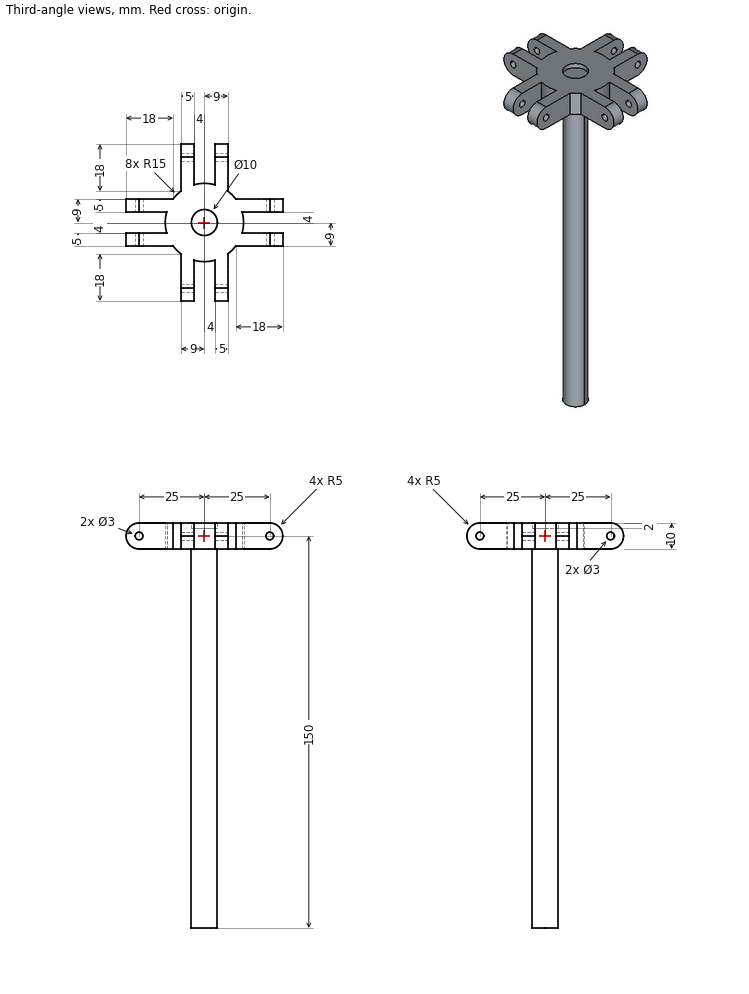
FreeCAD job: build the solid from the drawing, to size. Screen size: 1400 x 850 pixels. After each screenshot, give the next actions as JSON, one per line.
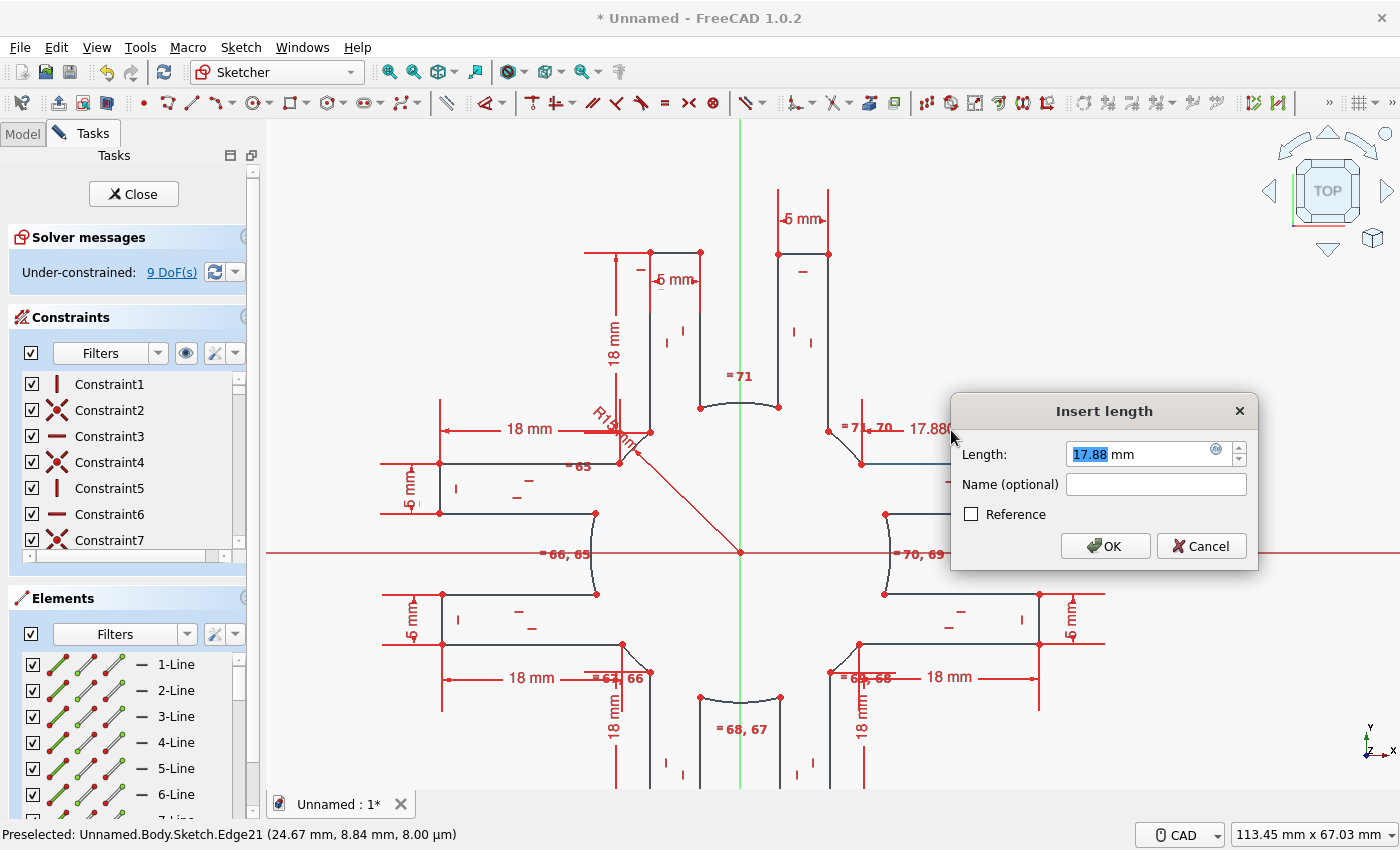
{"action": "type", "text": "18"}
{"action": "key", "text": "Return"}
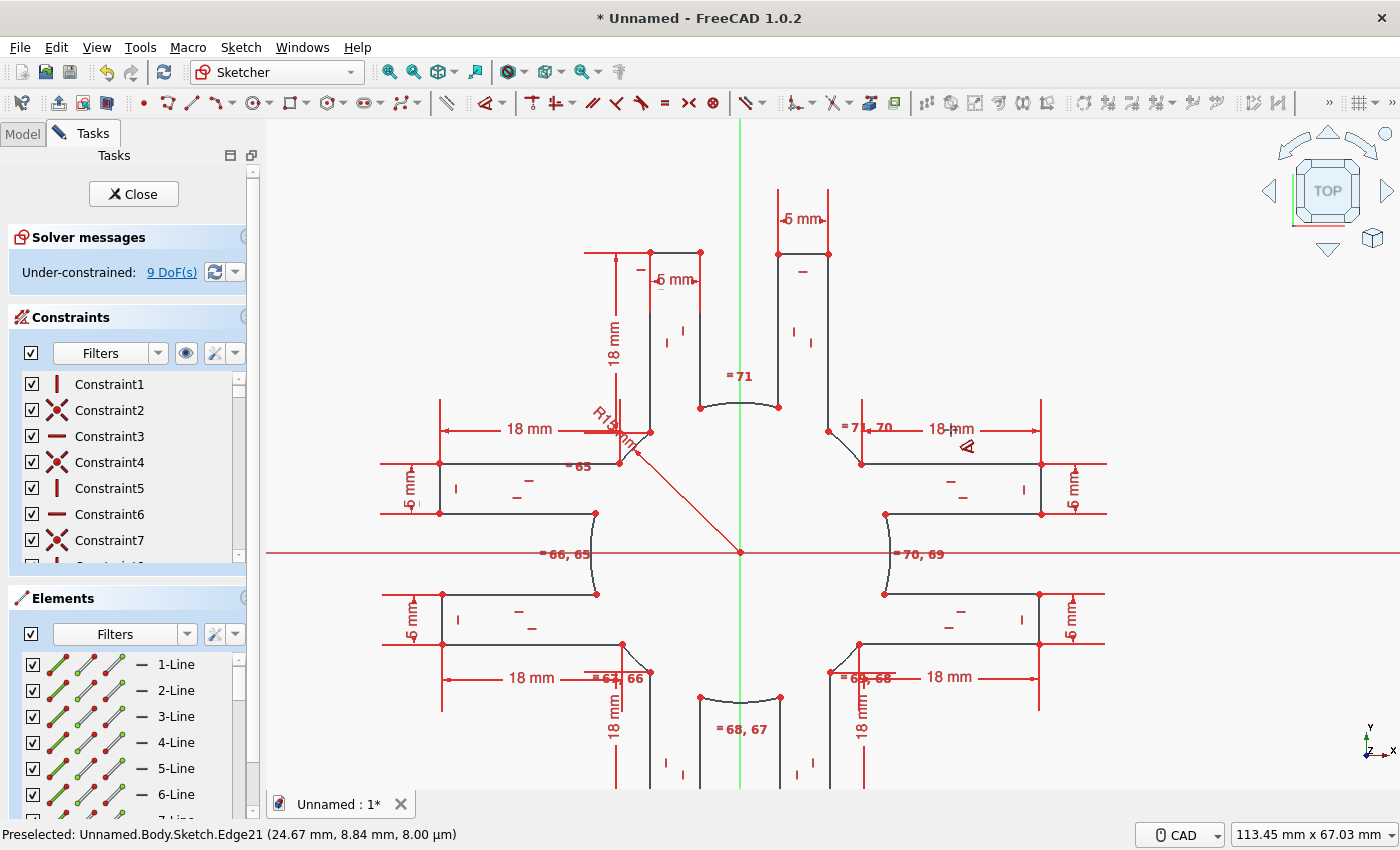
{"action": "left_click", "coordinate": [828, 378]}
{"action": "left_click", "coordinate": [862, 343]}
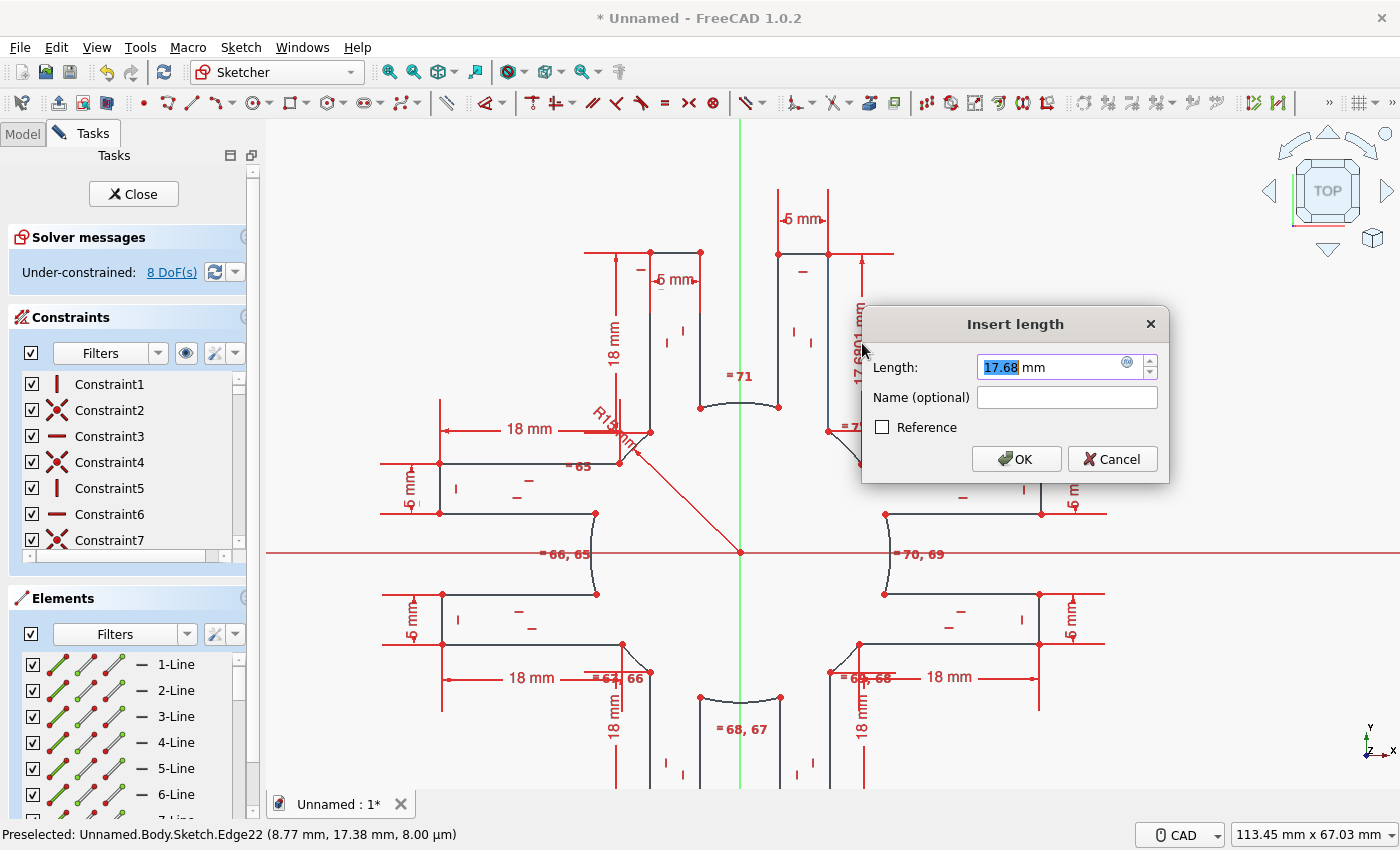
{"action": "type", "text": "18"}
{"action": "key", "text": "Return"}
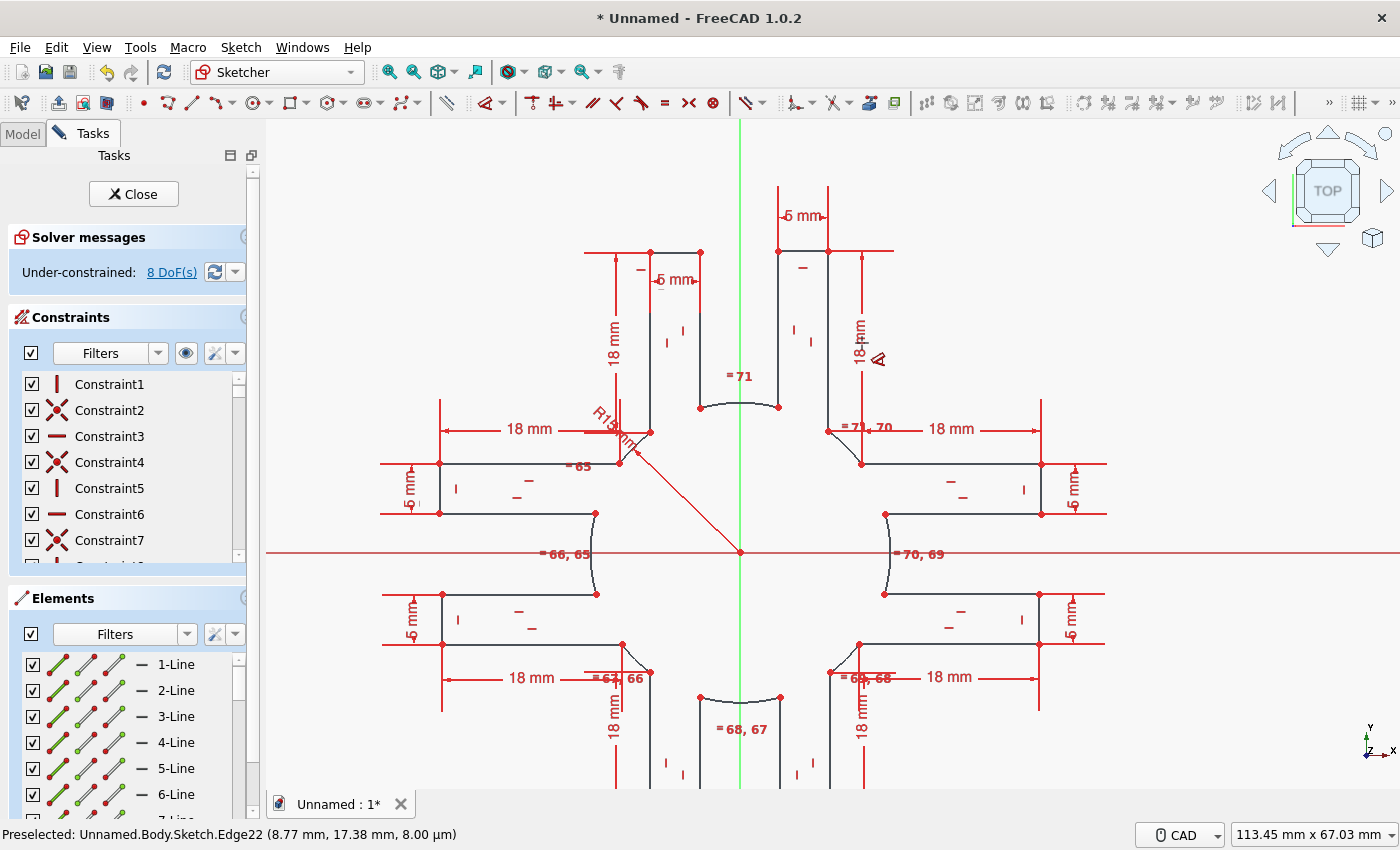
{"action": "left_click", "coordinate": [700, 408]}
{"action": "left_click", "coordinate": [720, 374]}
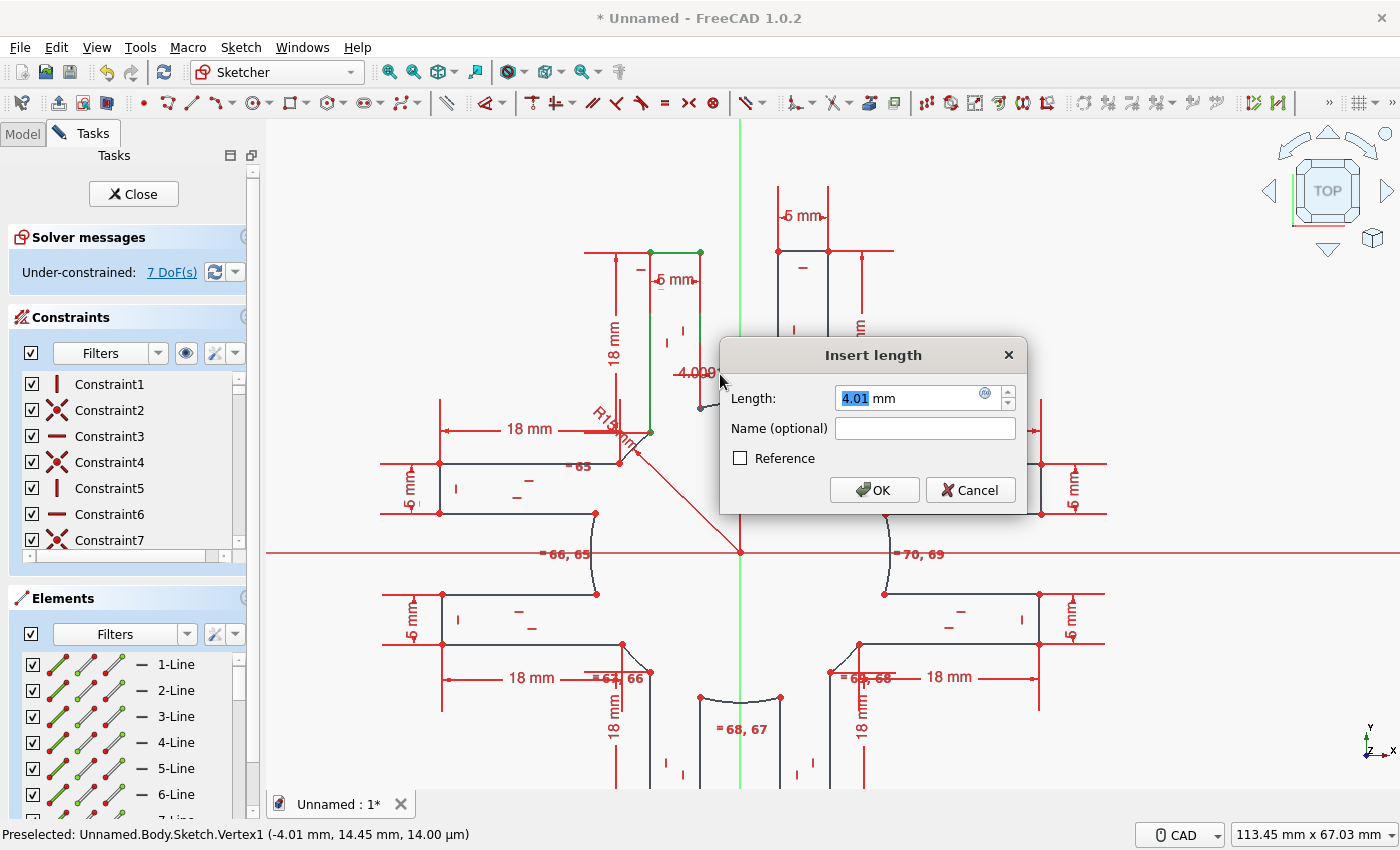
{"action": "type", "text": "4"}
{"action": "key", "text": "Return"}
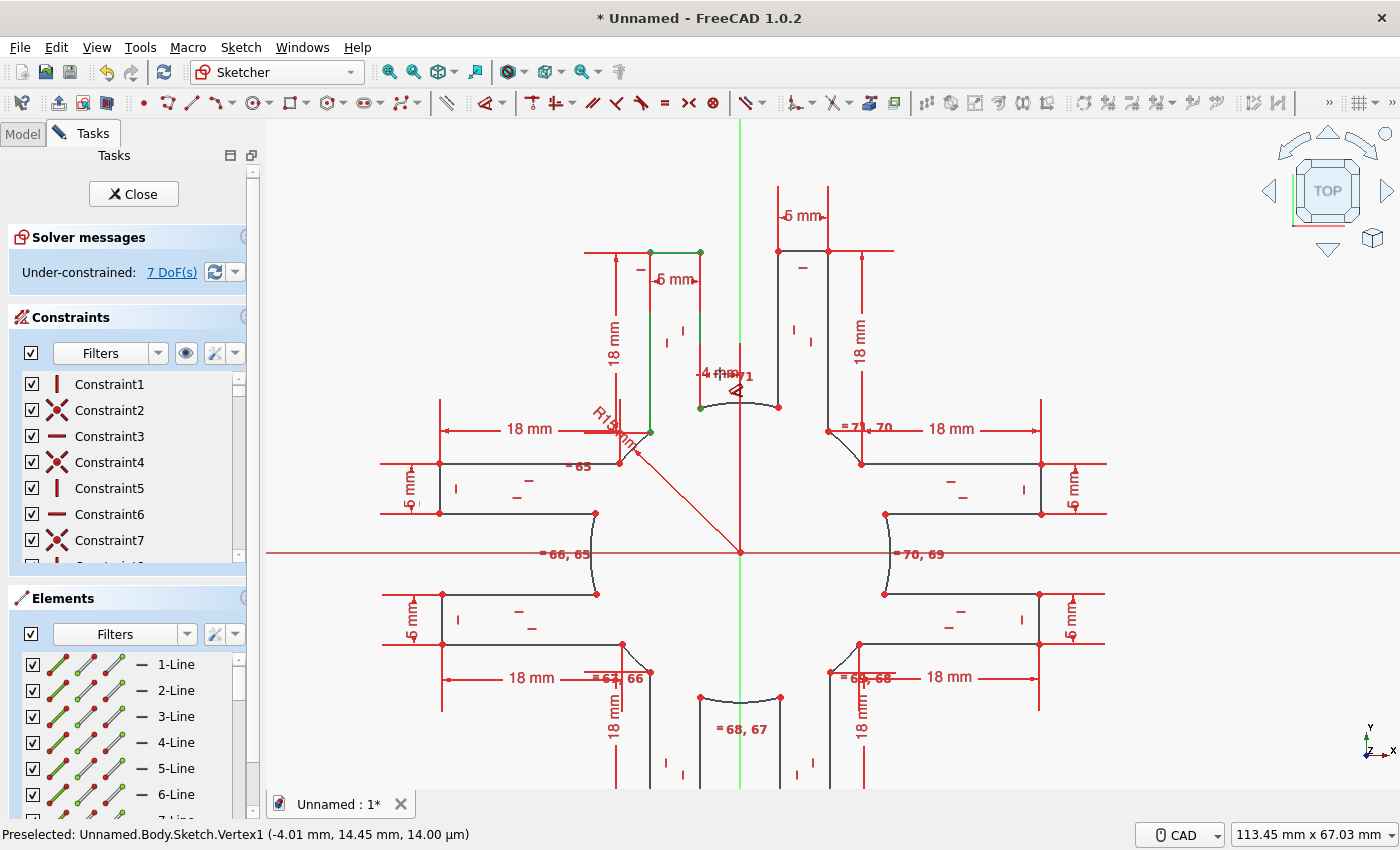
{"action": "left_click", "coordinate": [620, 464]}
{"action": "left_click", "coordinate": [586, 488]}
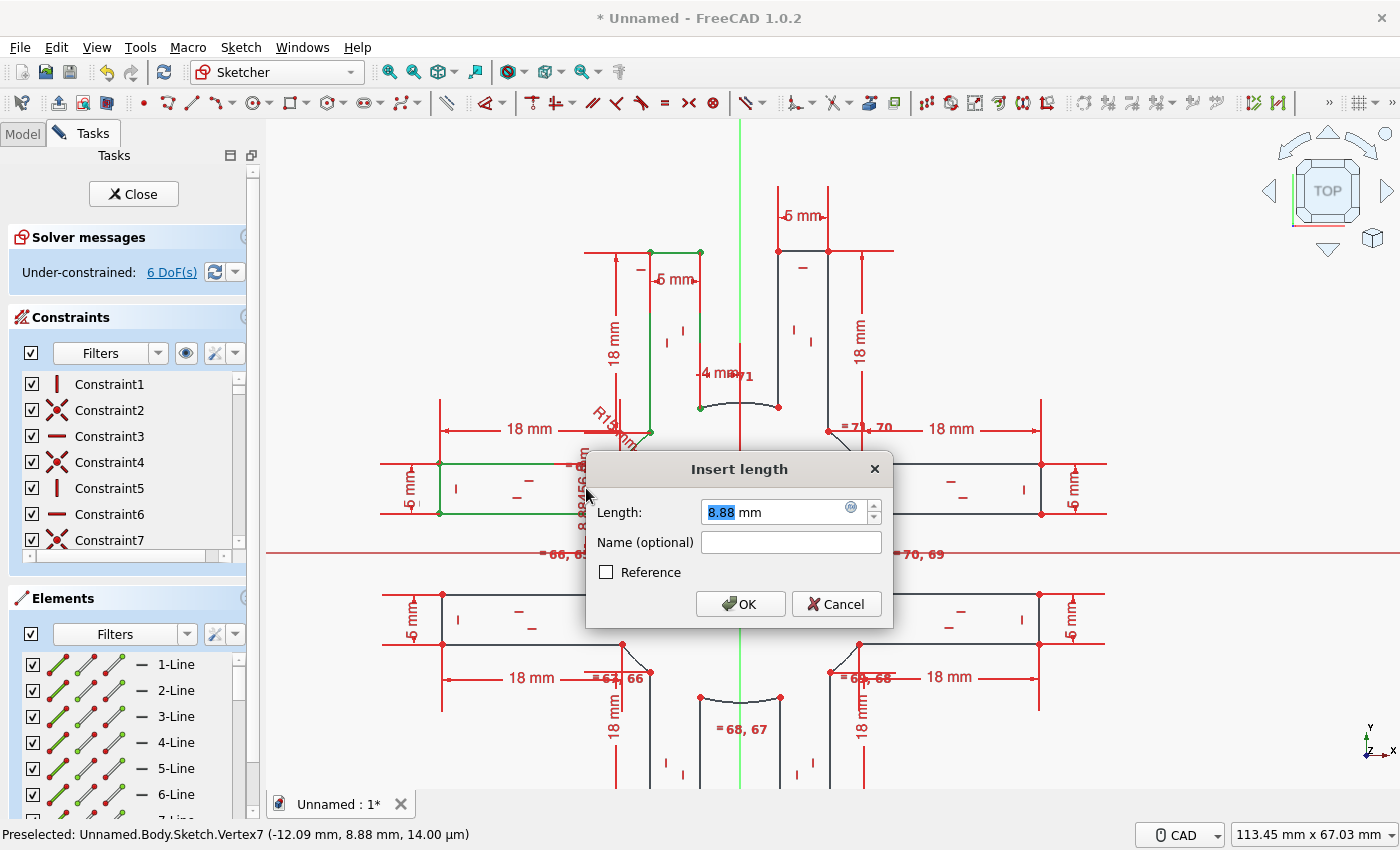
{"action": "type", "text": "9"}
{"action": "key", "text": "Return"}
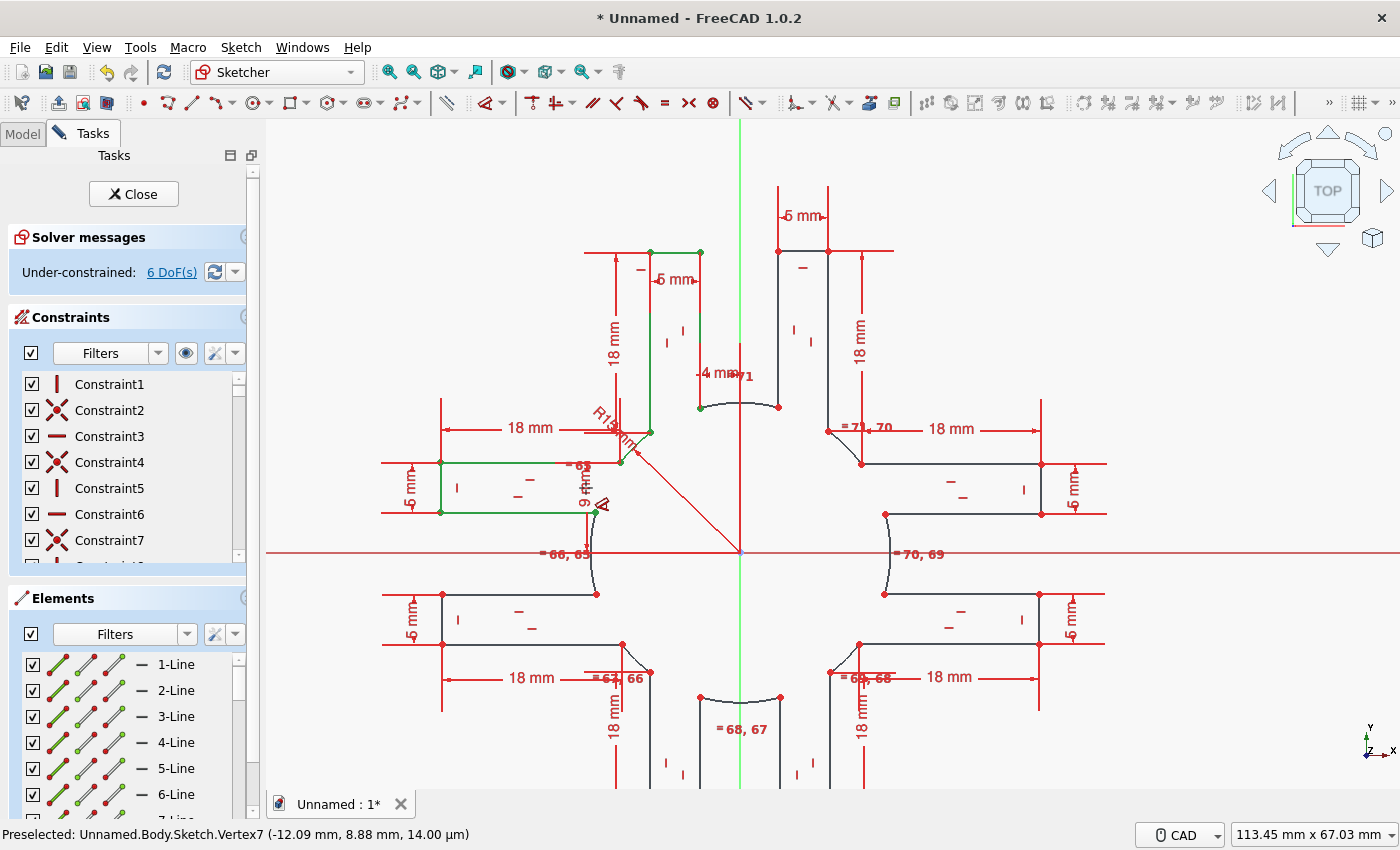
{"action": "left_click", "coordinate": [597, 595]}
{"action": "left_click", "coordinate": [563, 574]}